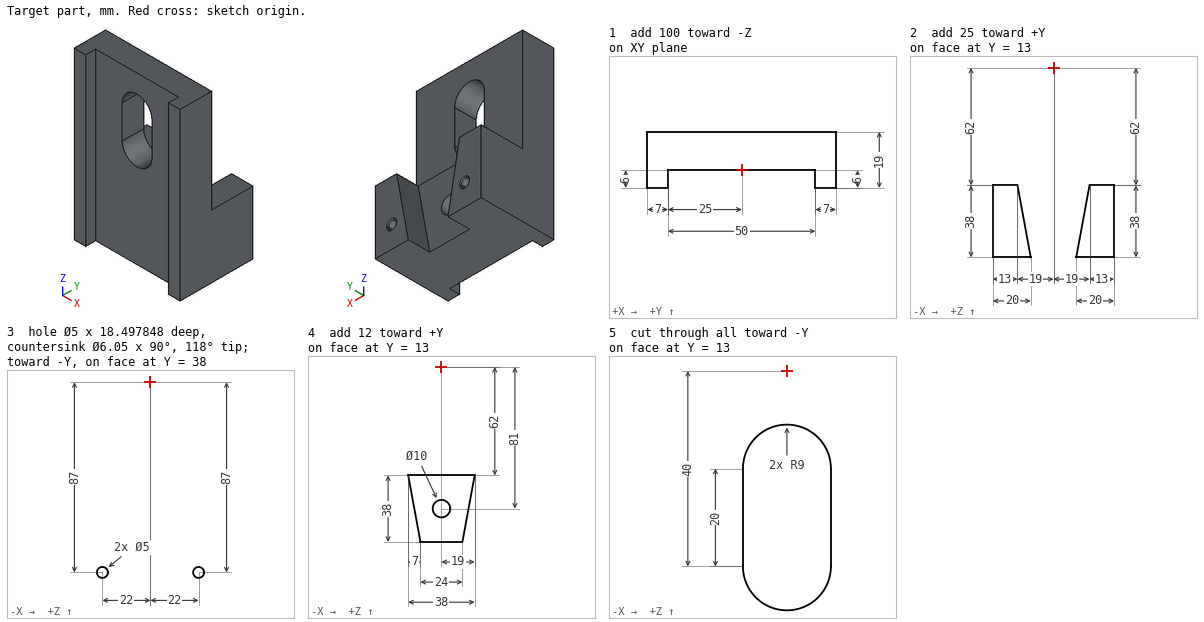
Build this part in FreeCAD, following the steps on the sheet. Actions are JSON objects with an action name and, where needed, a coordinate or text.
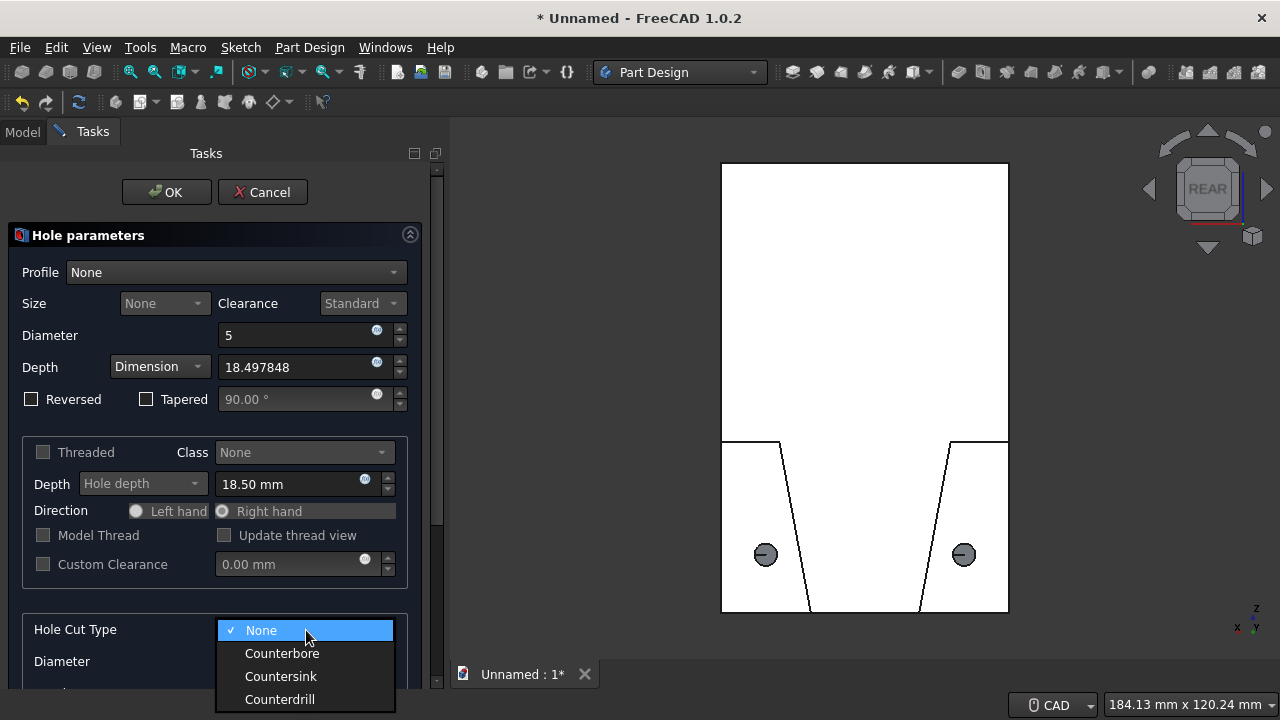
{"action": "left_click", "coordinate": [304, 676]}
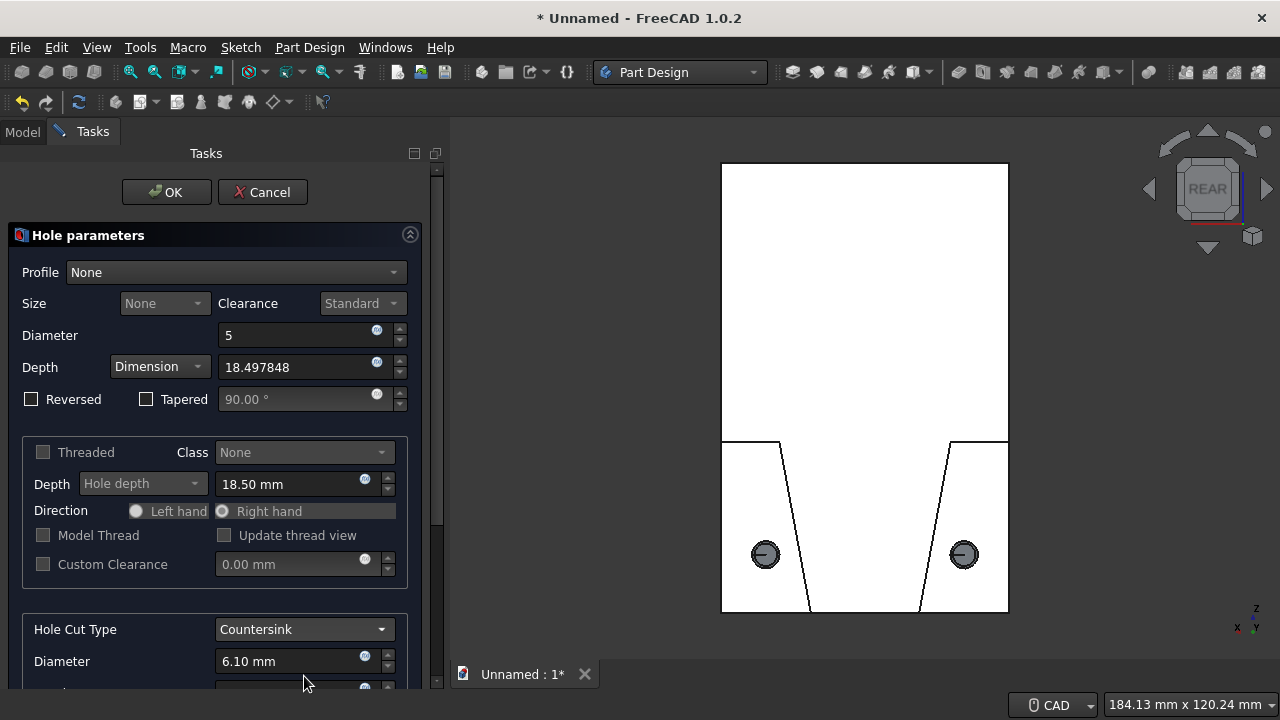
{"action": "triple_click", "coordinate": [298, 661]}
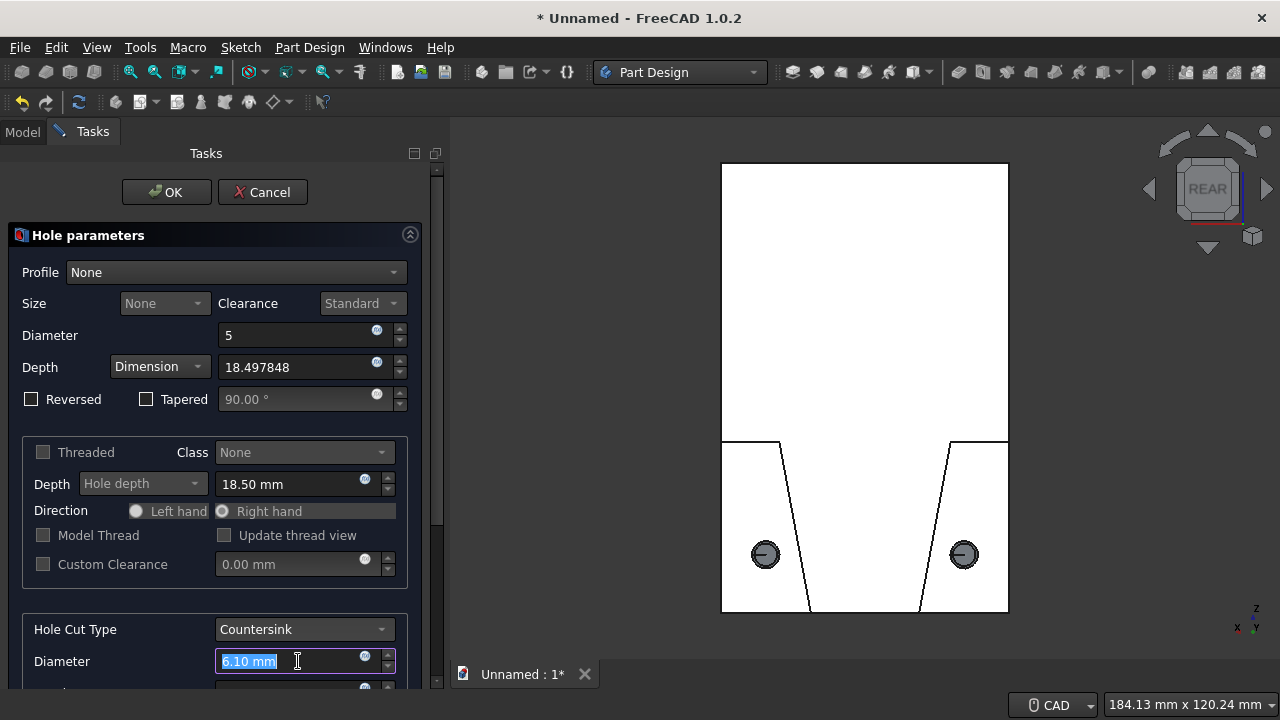
{"action": "type", "text": "6.05"}
{"action": "key", "text": "Tab"}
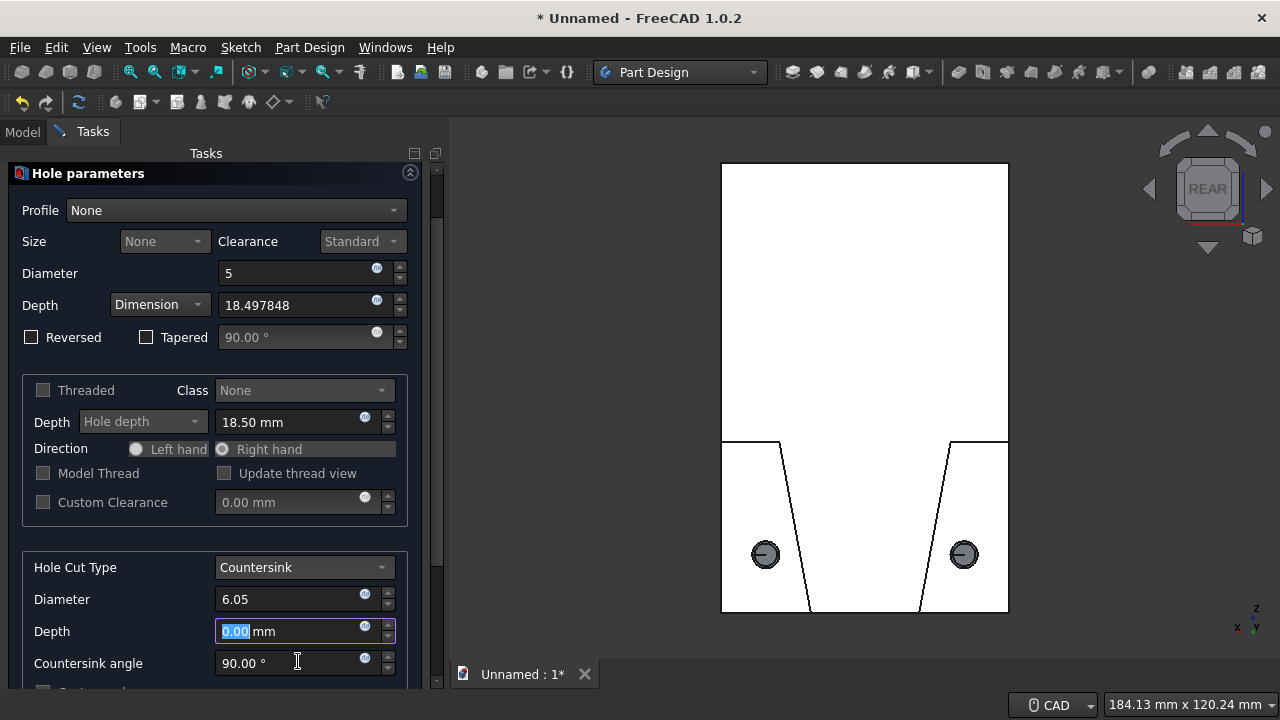
{"action": "scroll", "coordinate": [437, 426], "scroll_direction": "up", "scroll_amount": 2}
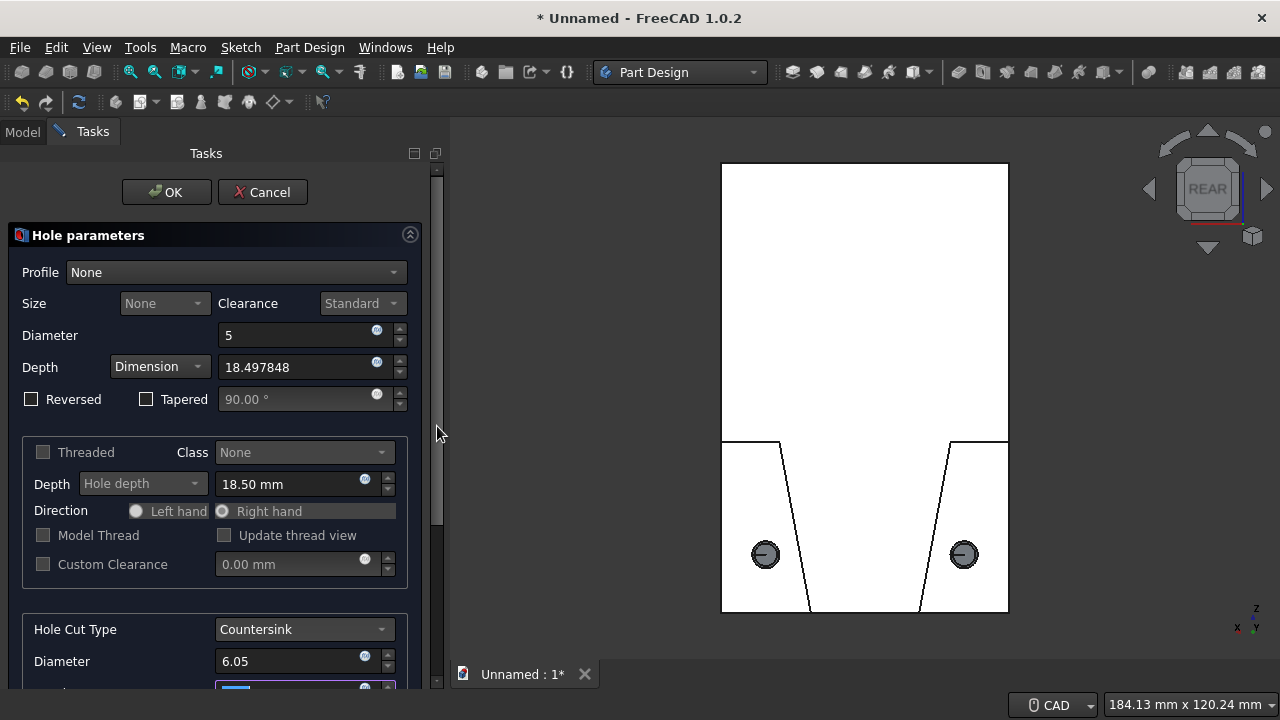
{"action": "left_click", "coordinate": [167, 192]}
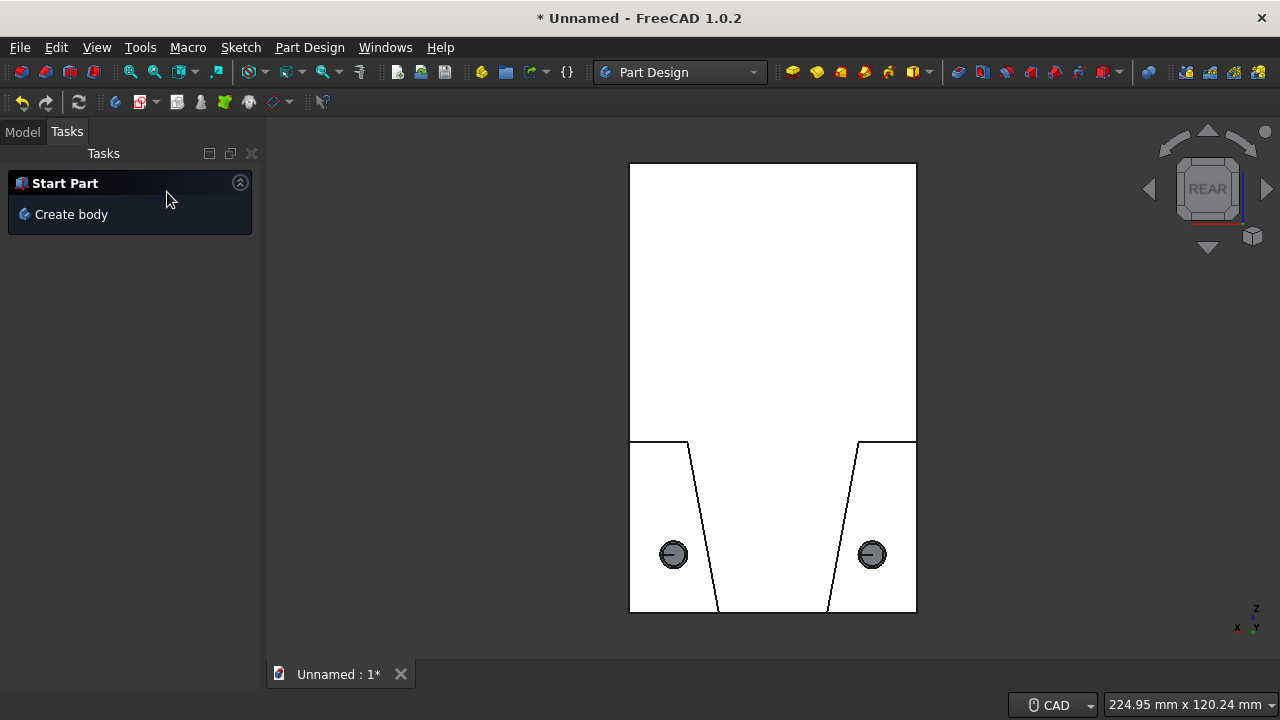
{"action": "left_click", "coordinate": [773, 323]}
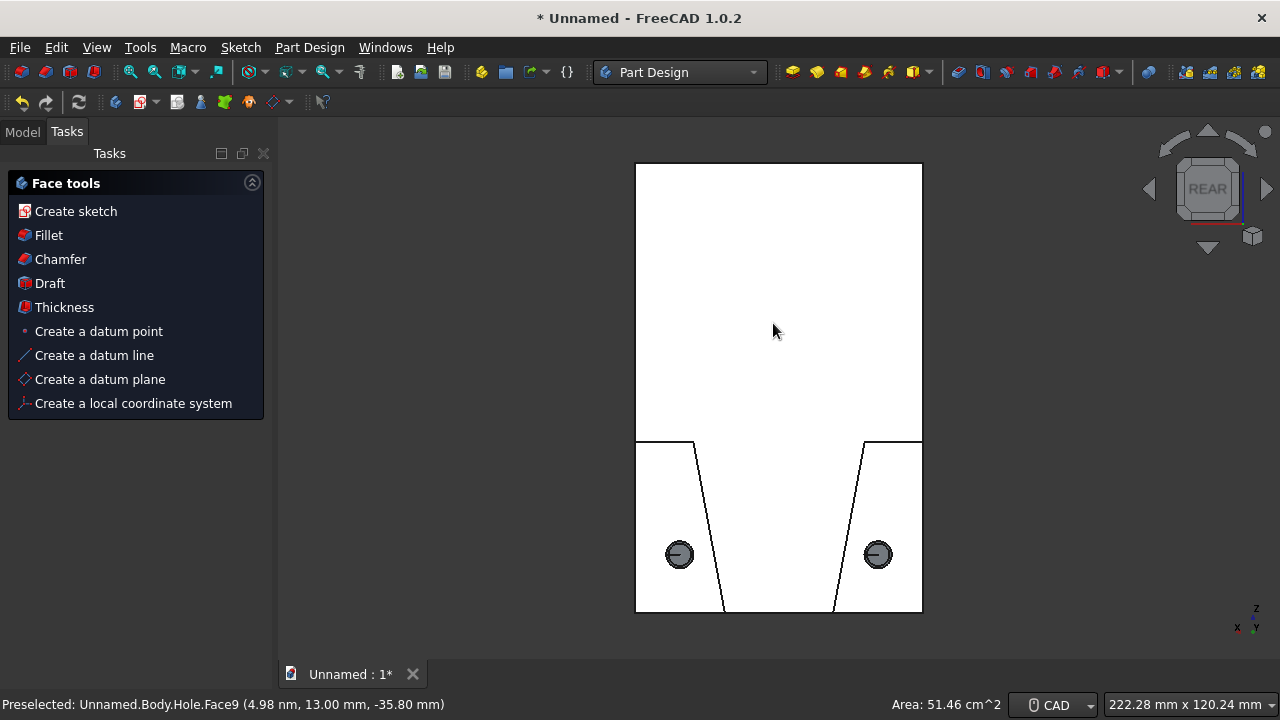
{"action": "left_click", "coordinate": [140, 102]}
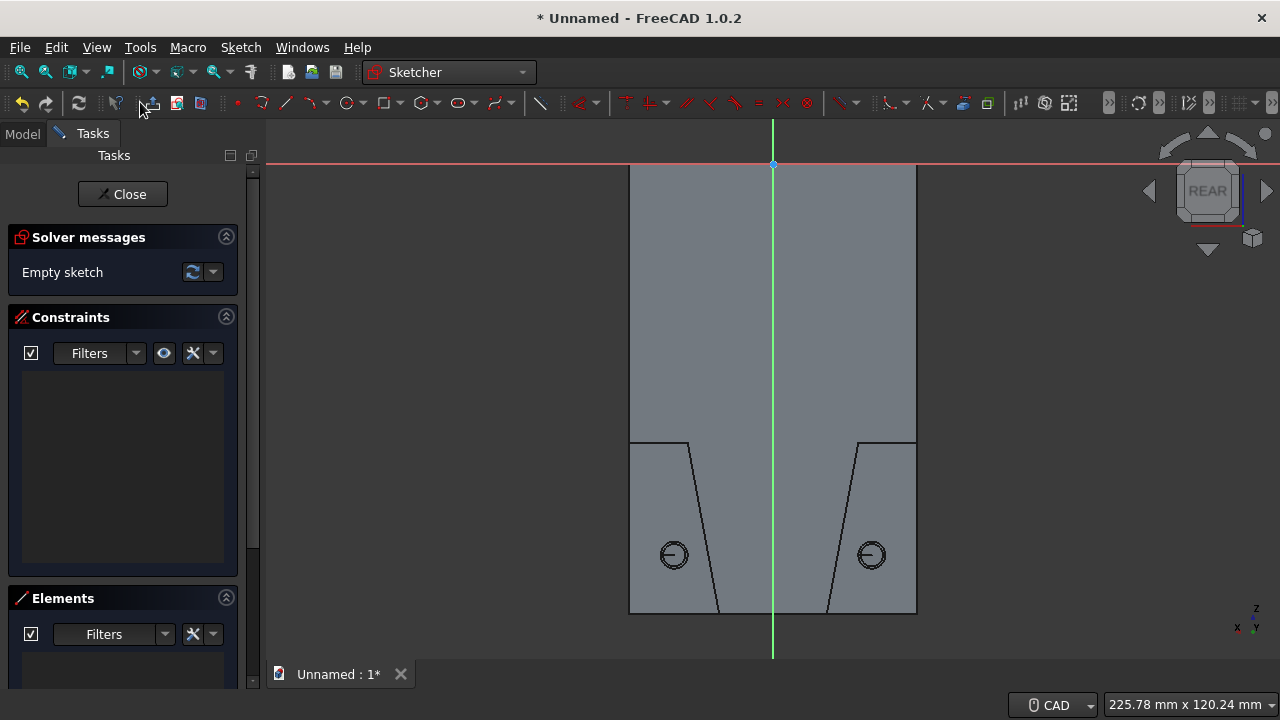
{"action": "key", "text": "q s"}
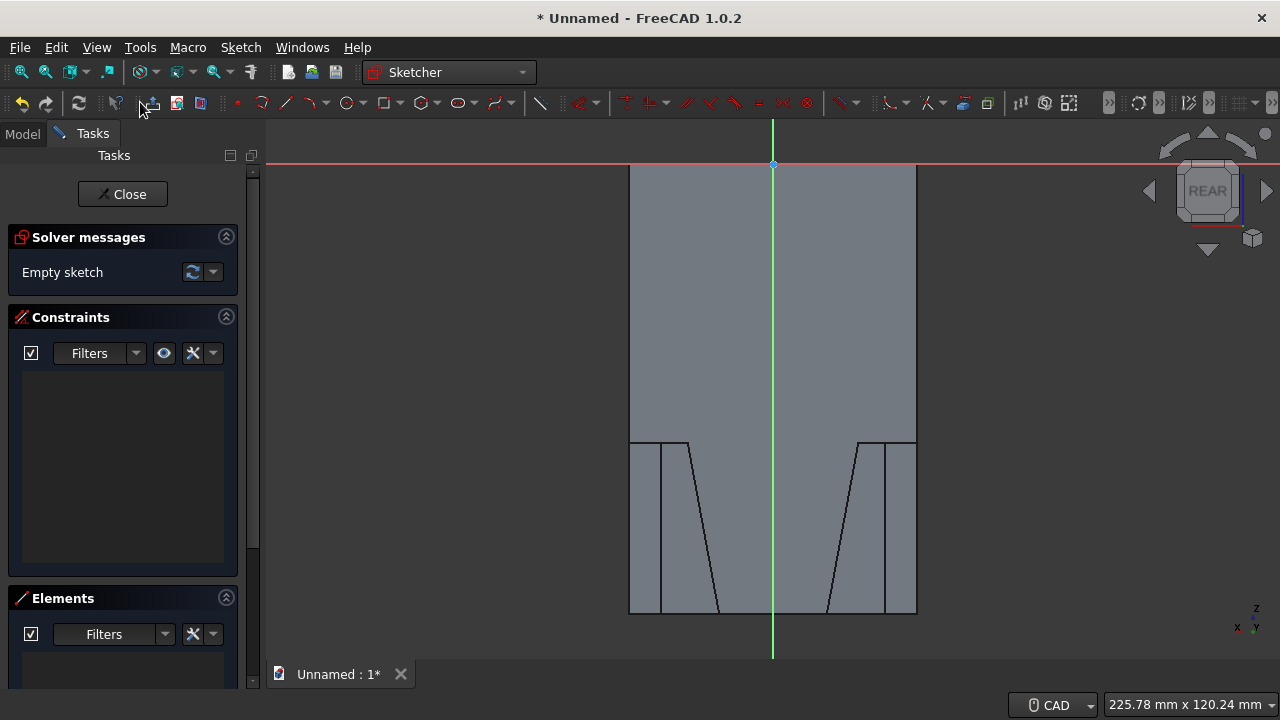
{"action": "scroll", "coordinate": [856, 631], "scroll_direction": "up", "scroll_amount": 3}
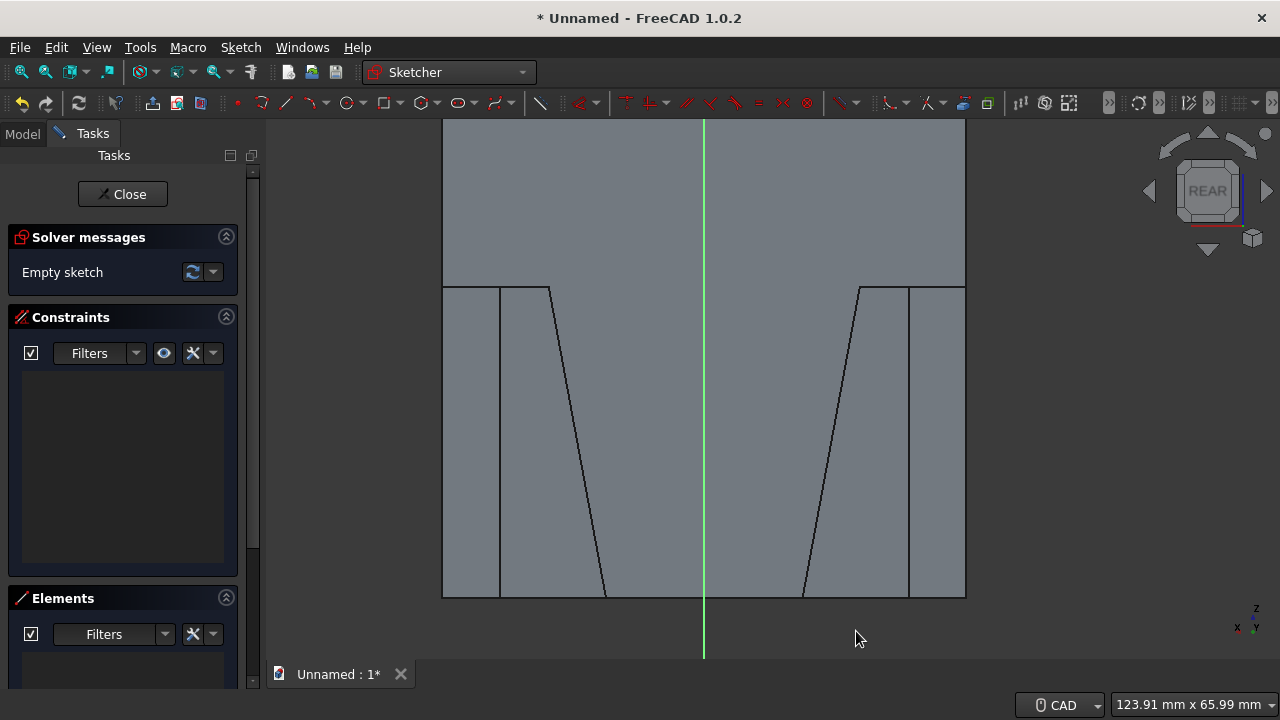
{"action": "key", "text": "g m"}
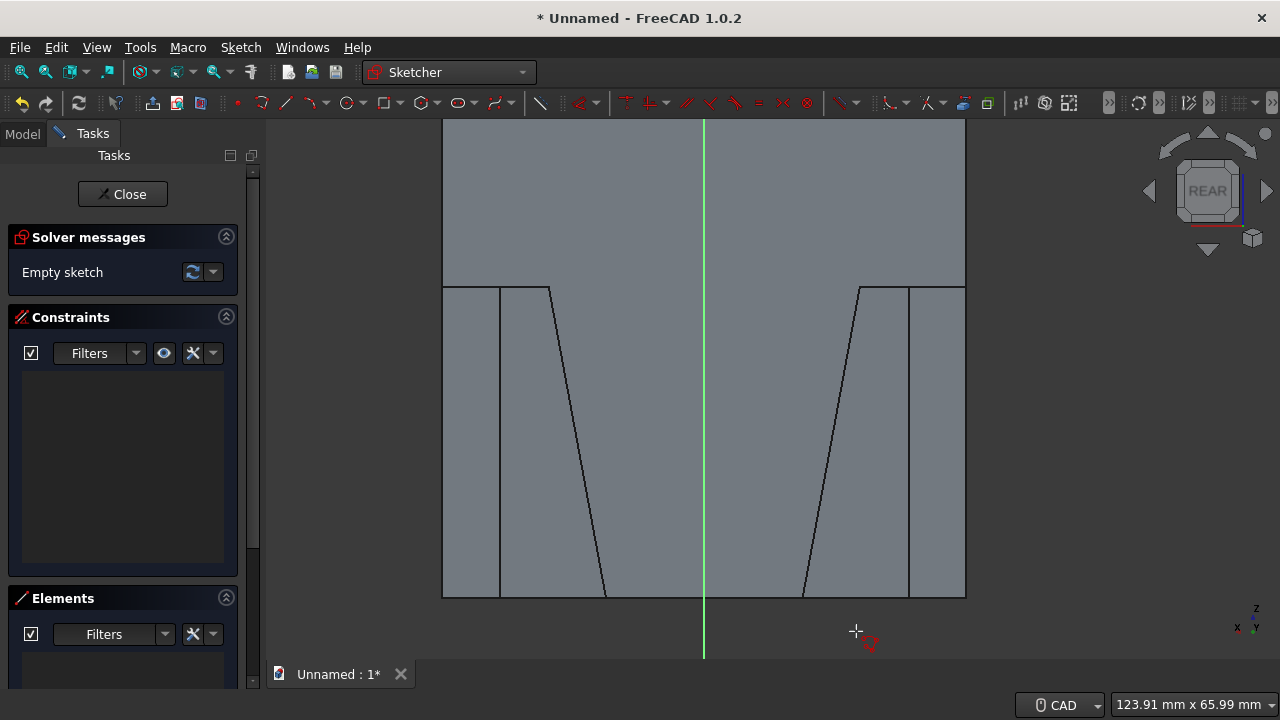
{"action": "left_click", "coordinate": [860, 287]}
{"action": "left_click", "coordinate": [549, 287]}
{"action": "left_click", "coordinate": [606, 598]}
{"action": "left_click", "coordinate": [802, 598]}
{"action": "left_click", "coordinate": [860, 288]}